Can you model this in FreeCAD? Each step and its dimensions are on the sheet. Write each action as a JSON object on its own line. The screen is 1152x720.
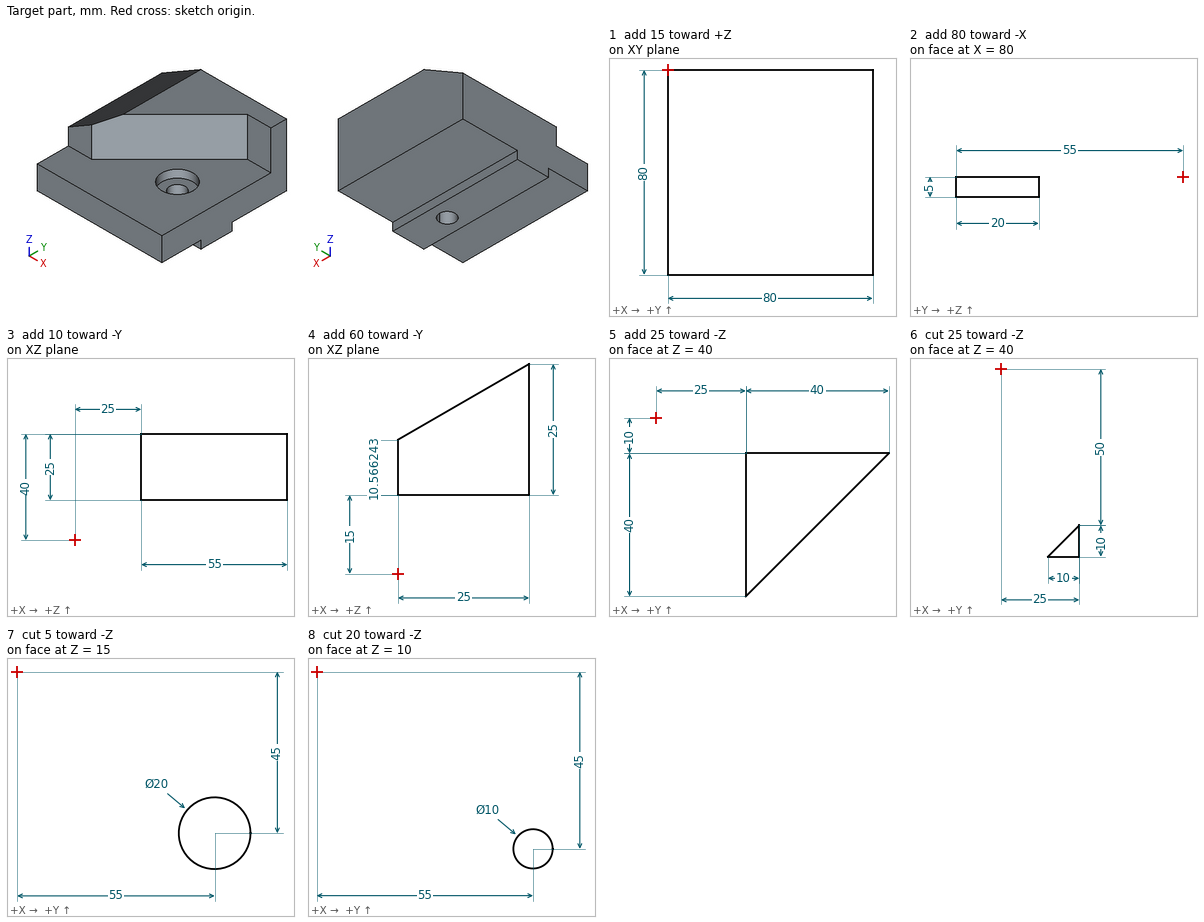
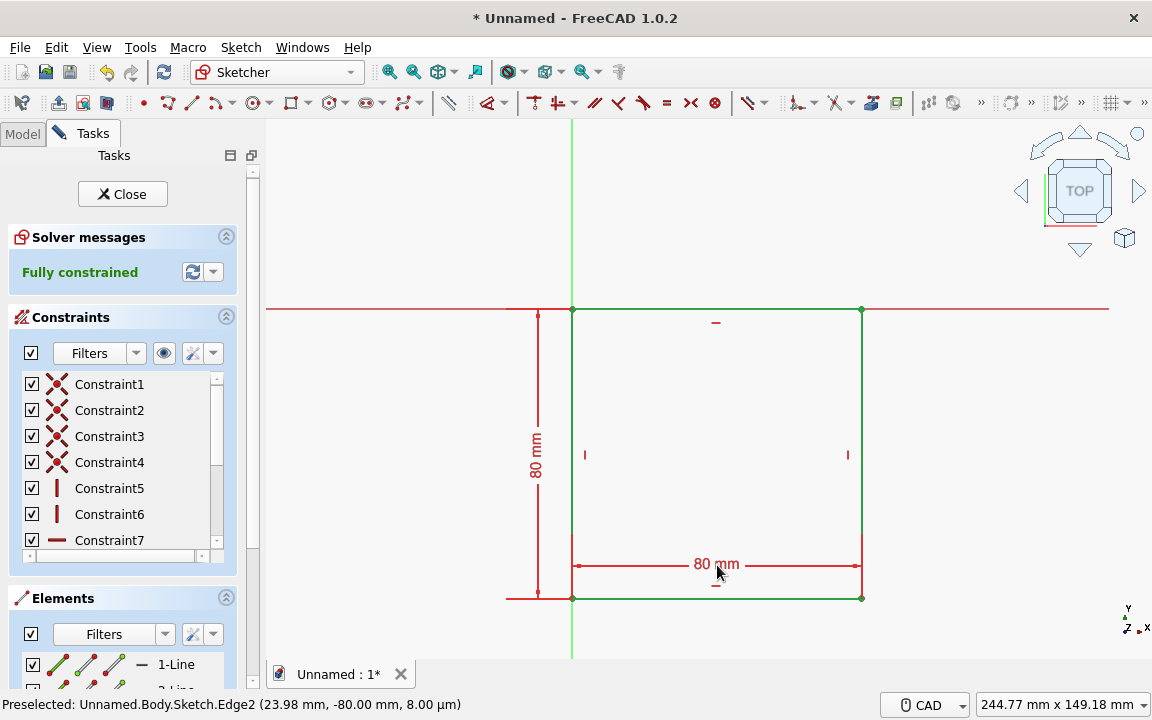
{"action": "left_click", "coordinate": [123, 194]}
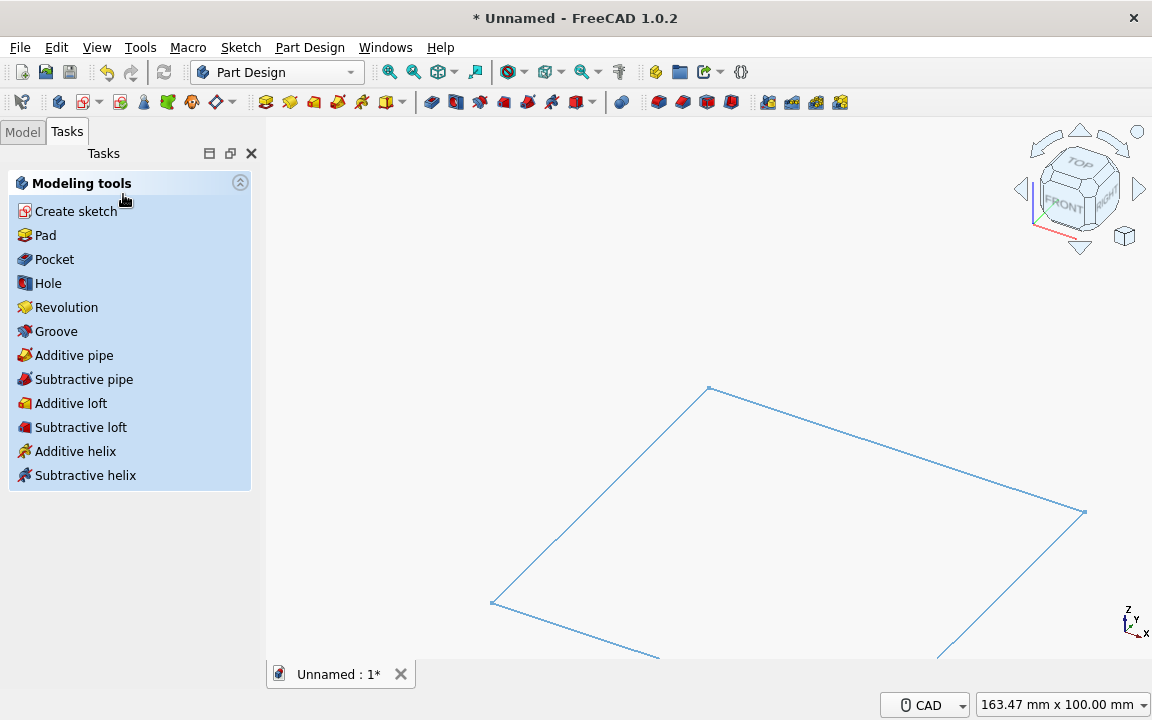
{"action": "left_click", "coordinate": [266, 102]}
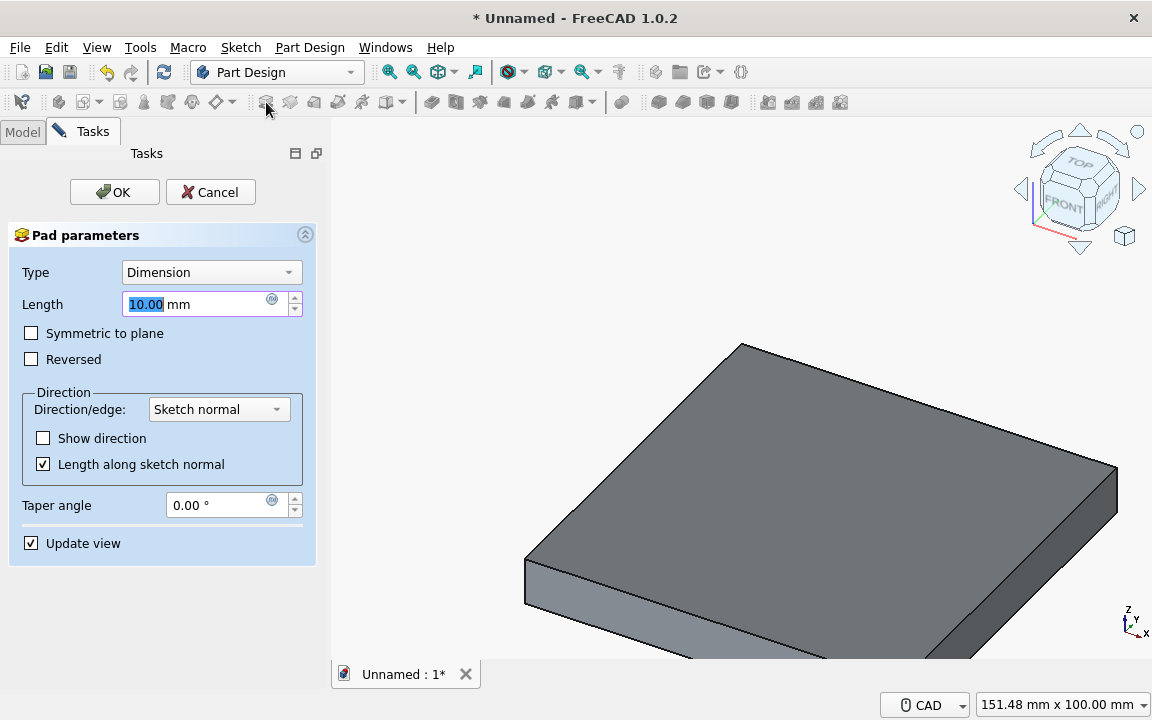
{"action": "type", "text": "15"}
{"action": "key", "text": "Tab"}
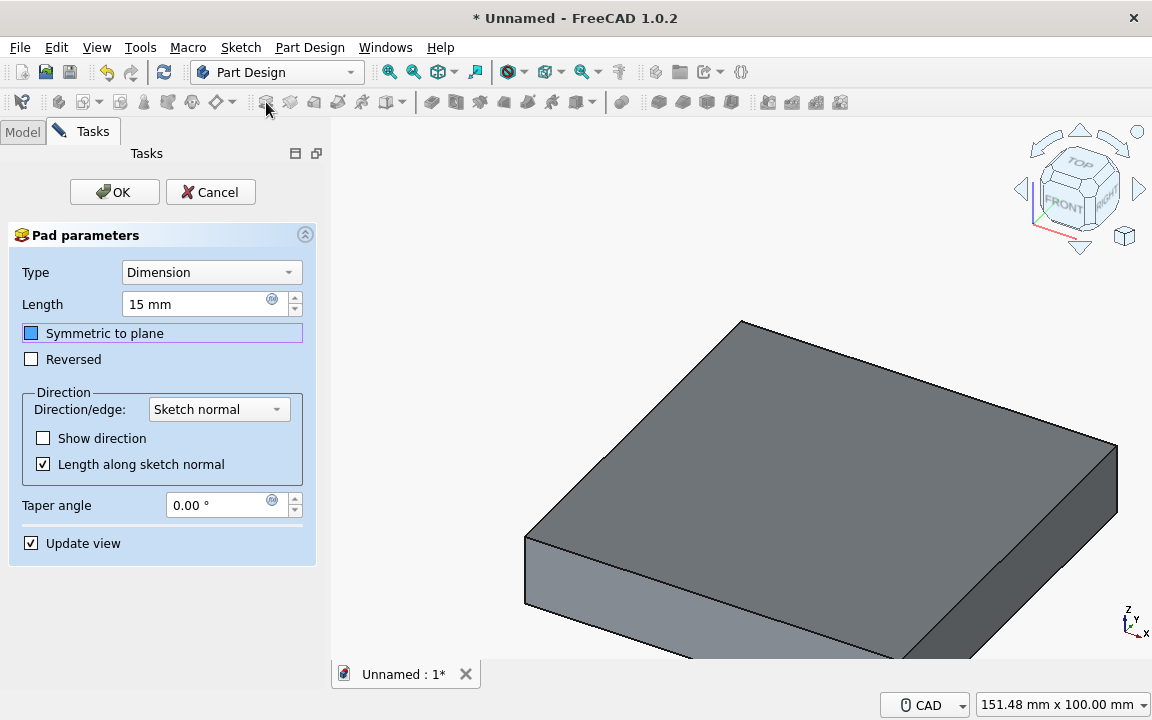
{"action": "left_click", "coordinate": [115, 192]}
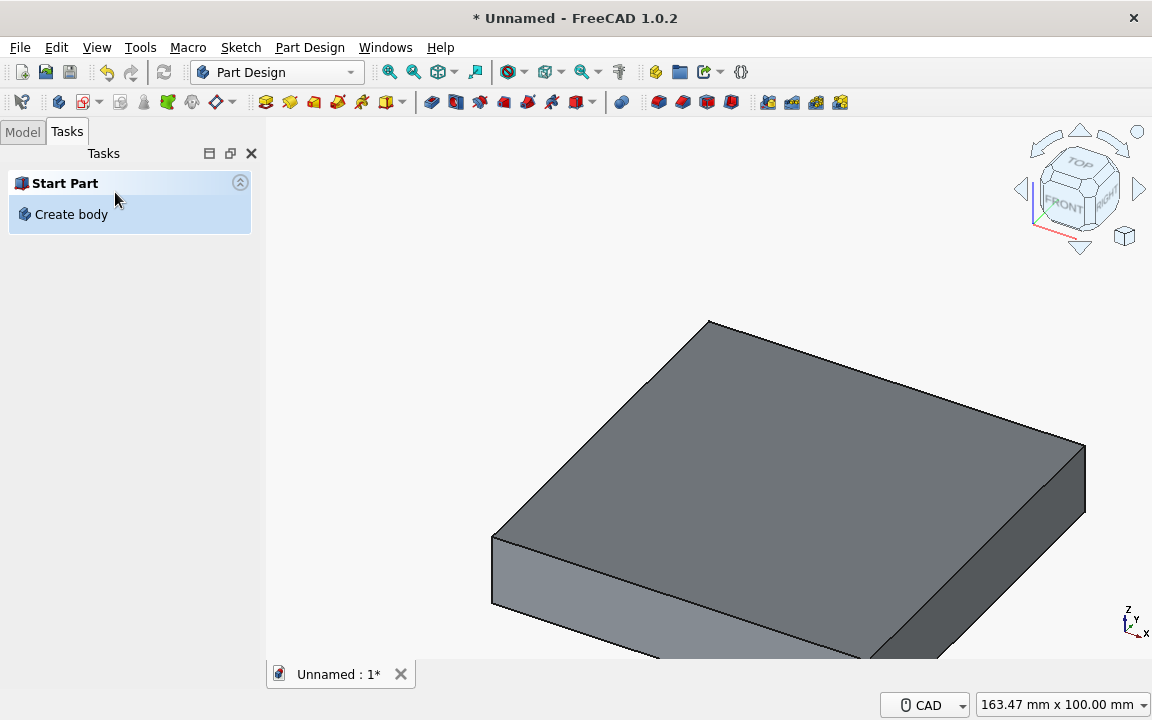
{"action": "left_click", "coordinate": [390, 72]}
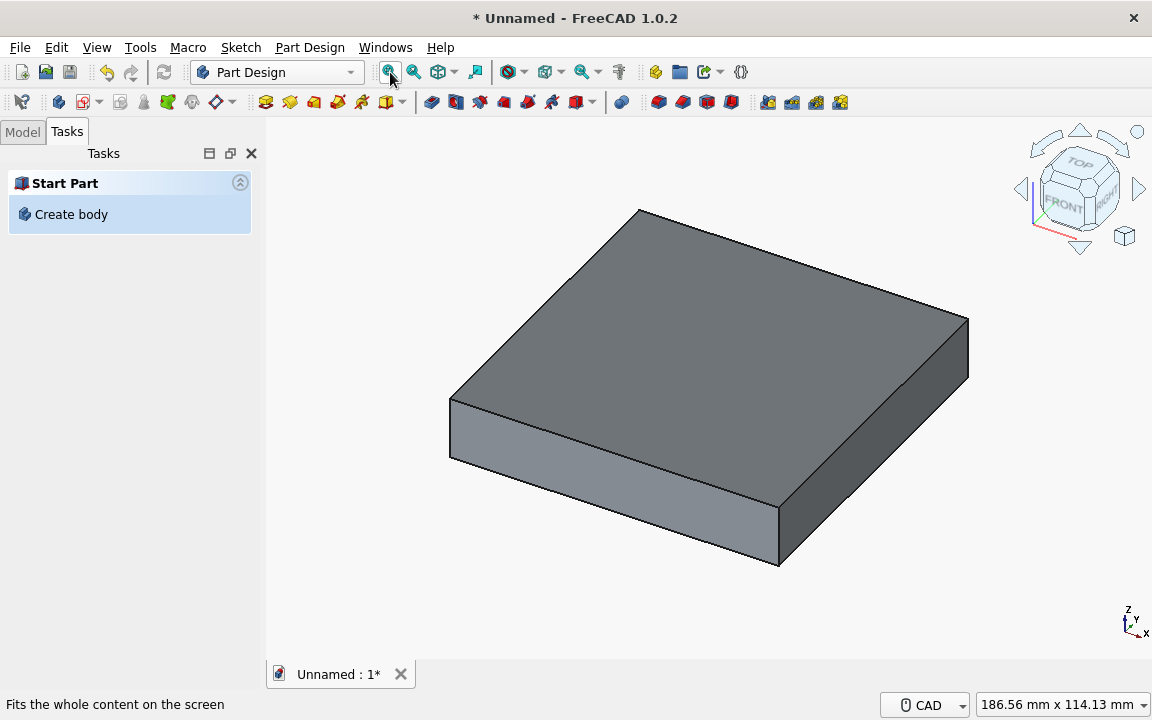
{"action": "left_click", "coordinate": [928, 388]}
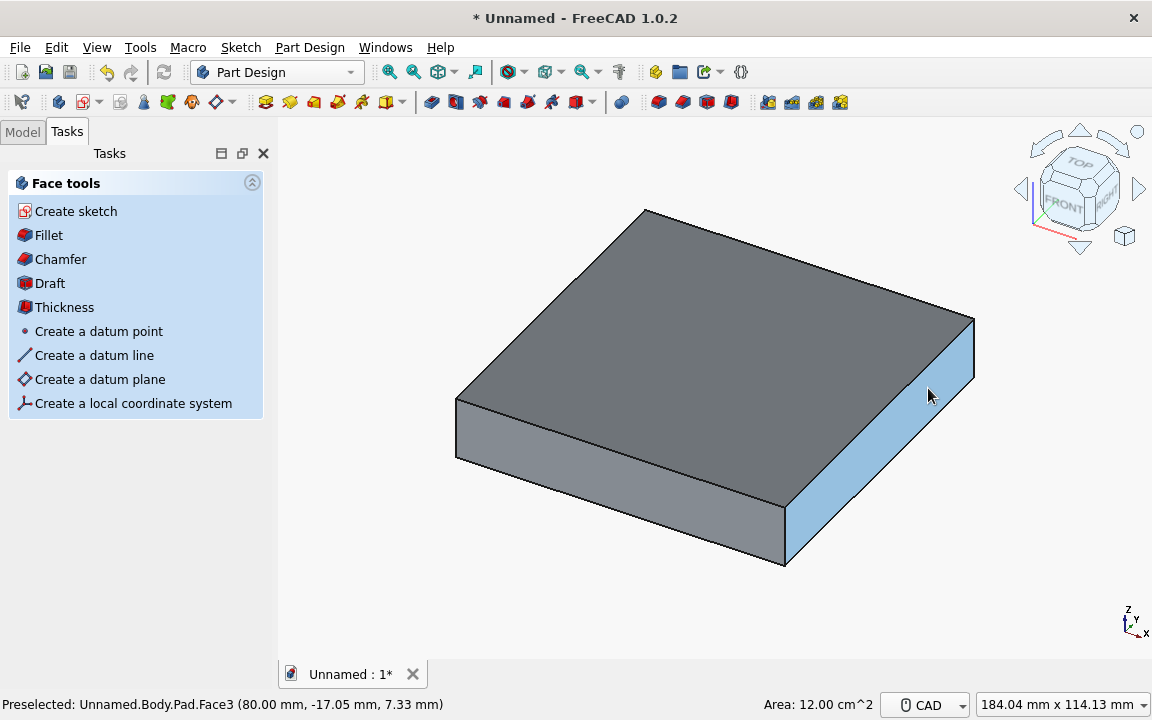
{"action": "left_click", "coordinate": [84, 102]}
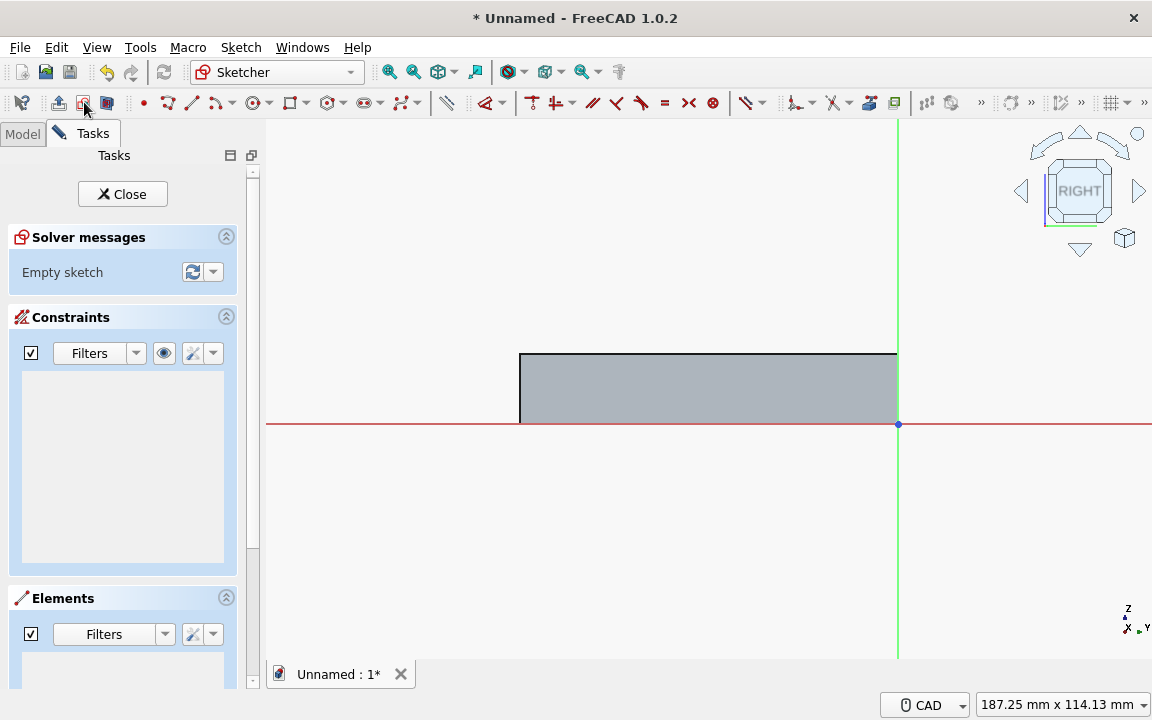
{"action": "scroll", "coordinate": [697, 448], "scroll_direction": "up", "scroll_amount": 8}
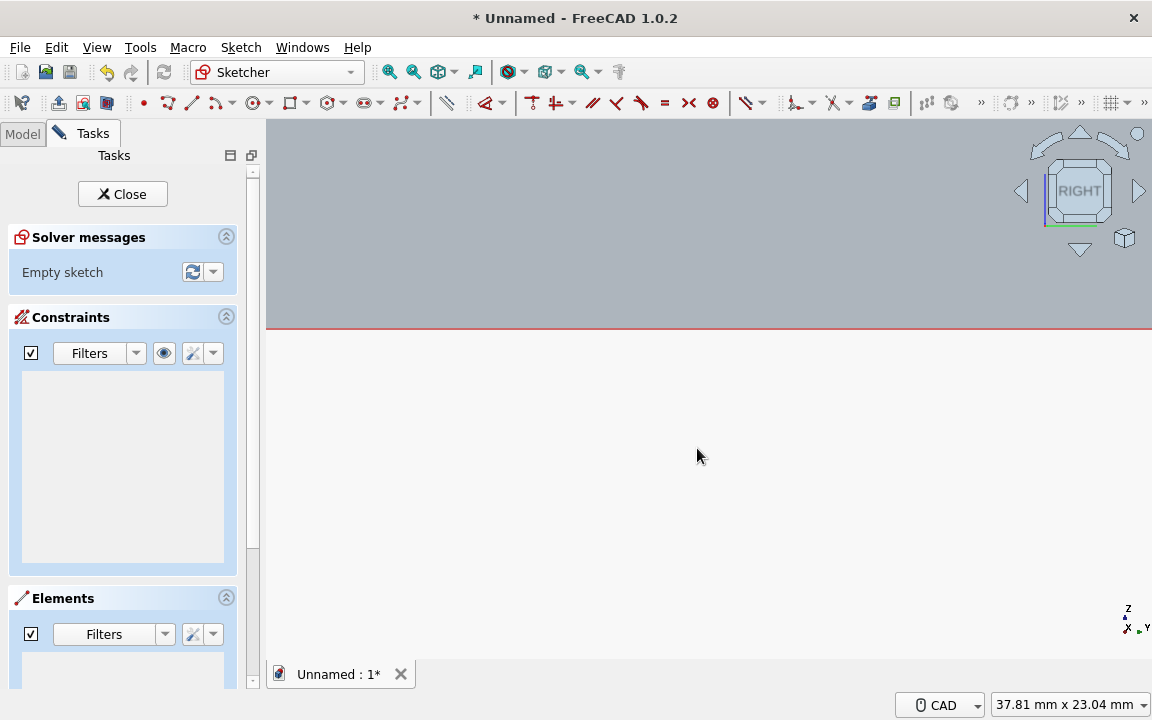
{"action": "left_click", "coordinate": [290, 104]}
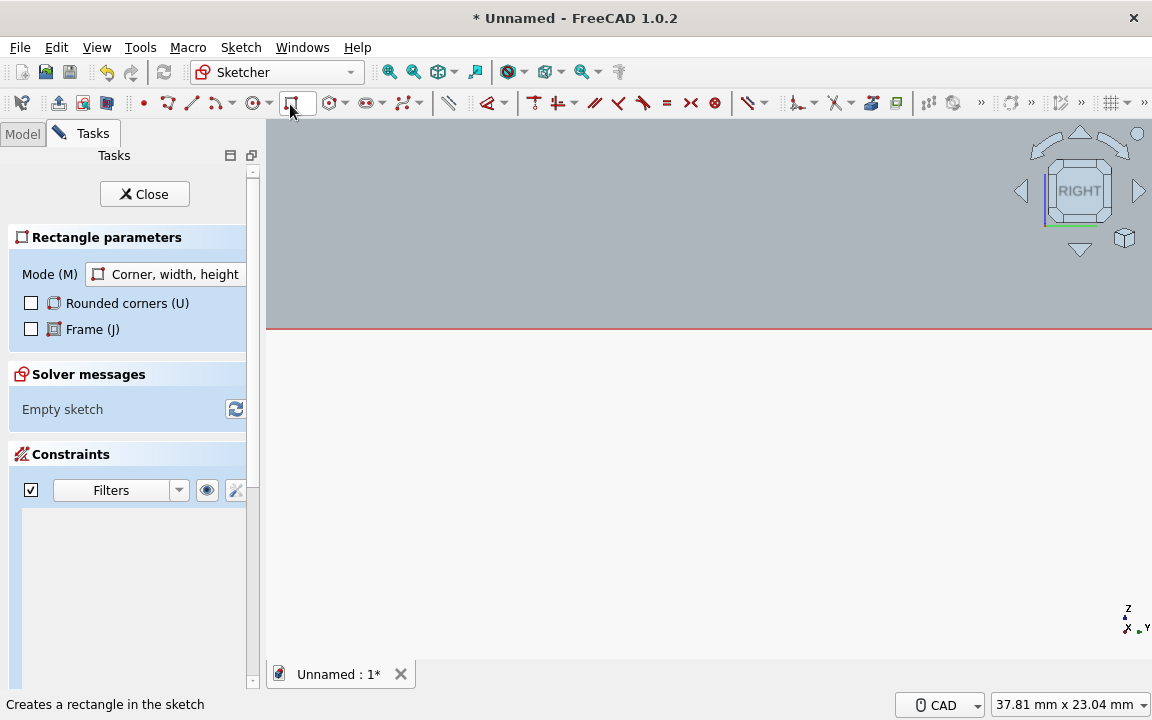
{"action": "left_click", "coordinate": [403, 329]}
{"action": "left_click", "coordinate": [872, 446]}
{"action": "key", "text": "Escape"}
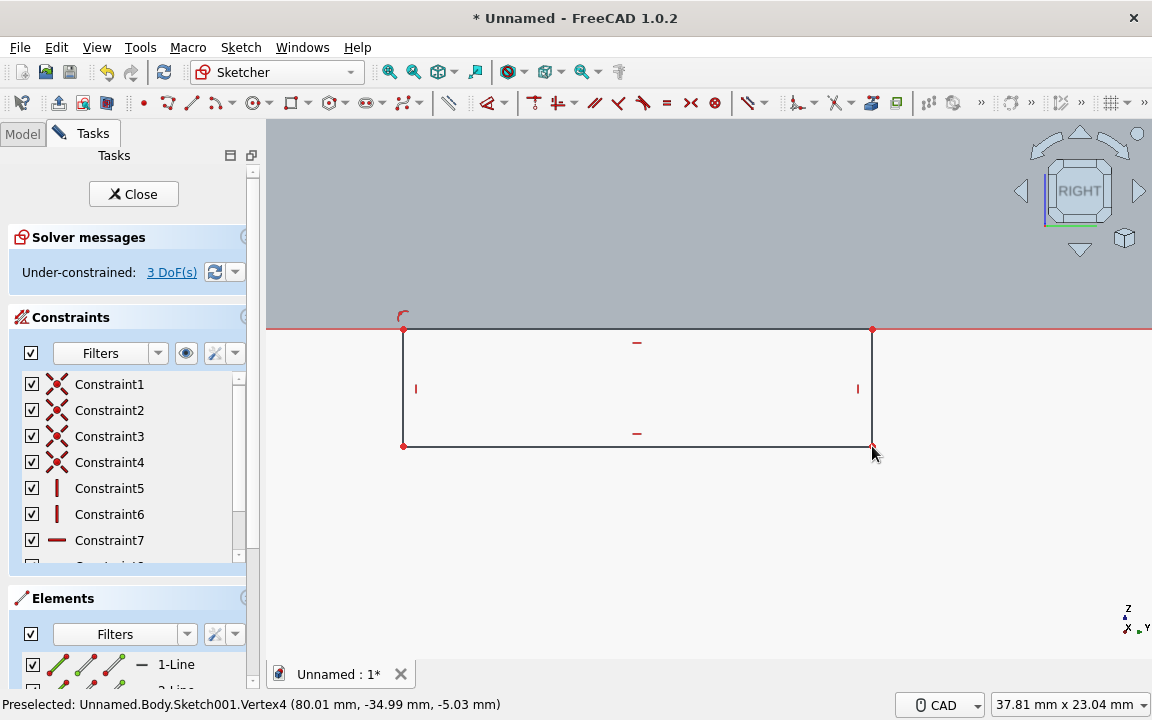
{"action": "left_click", "coordinate": [488, 104]}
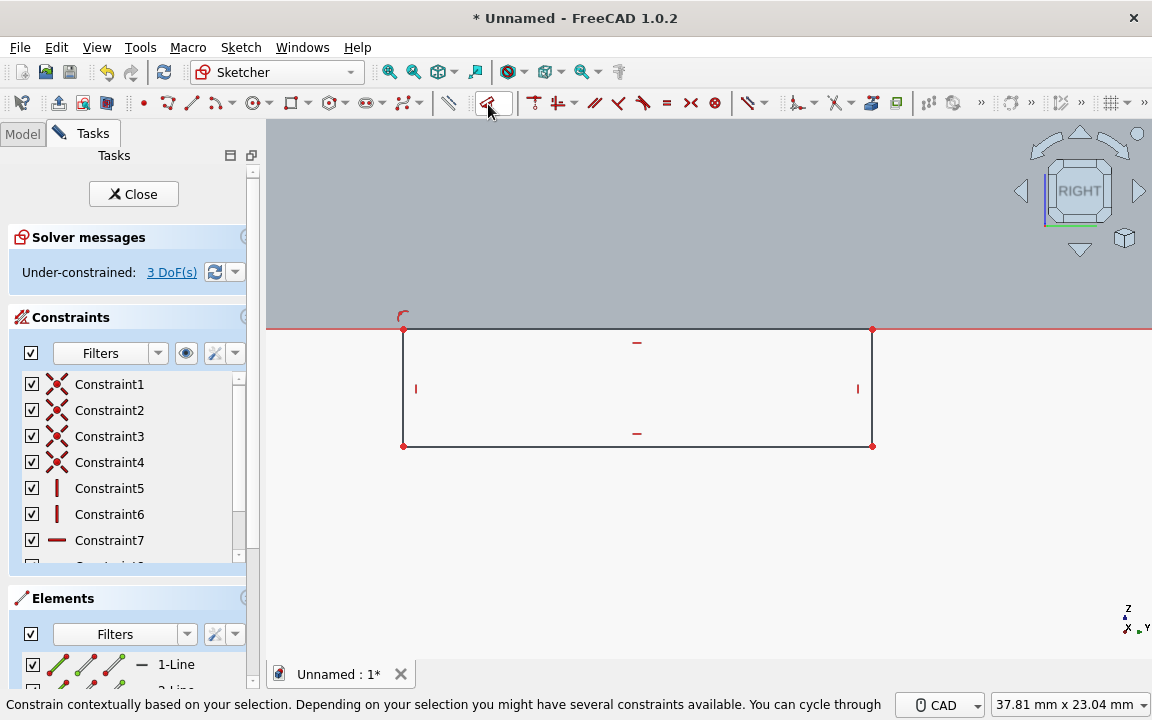
{"action": "left_click", "coordinate": [403, 364]}
{"action": "left_click", "coordinate": [369, 388]}